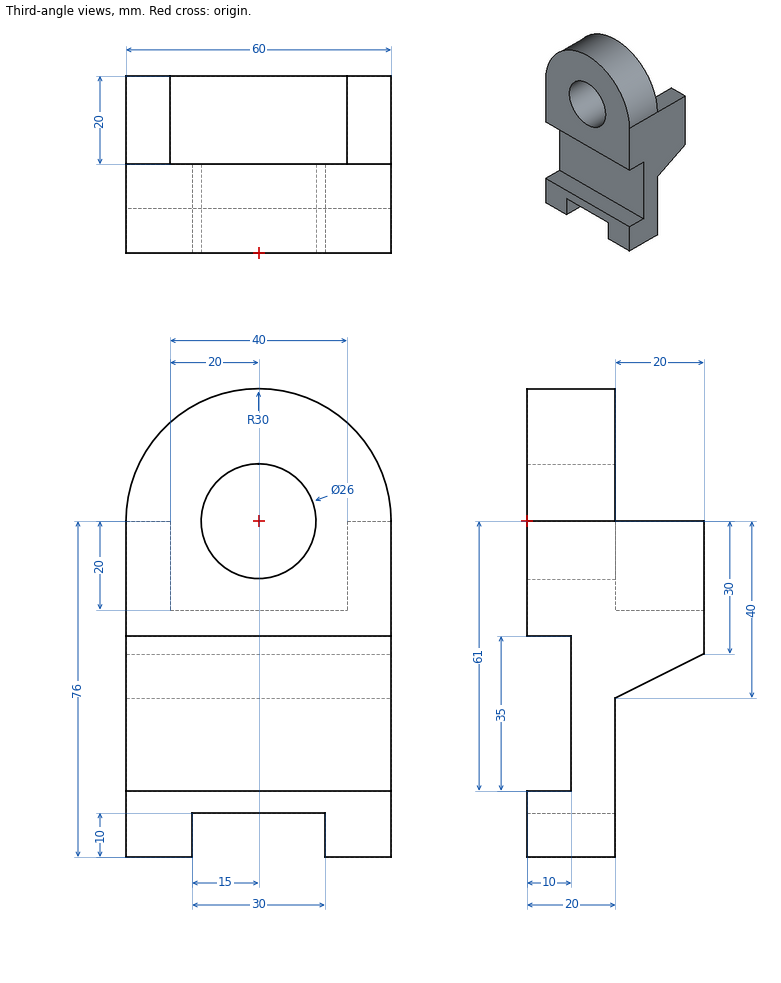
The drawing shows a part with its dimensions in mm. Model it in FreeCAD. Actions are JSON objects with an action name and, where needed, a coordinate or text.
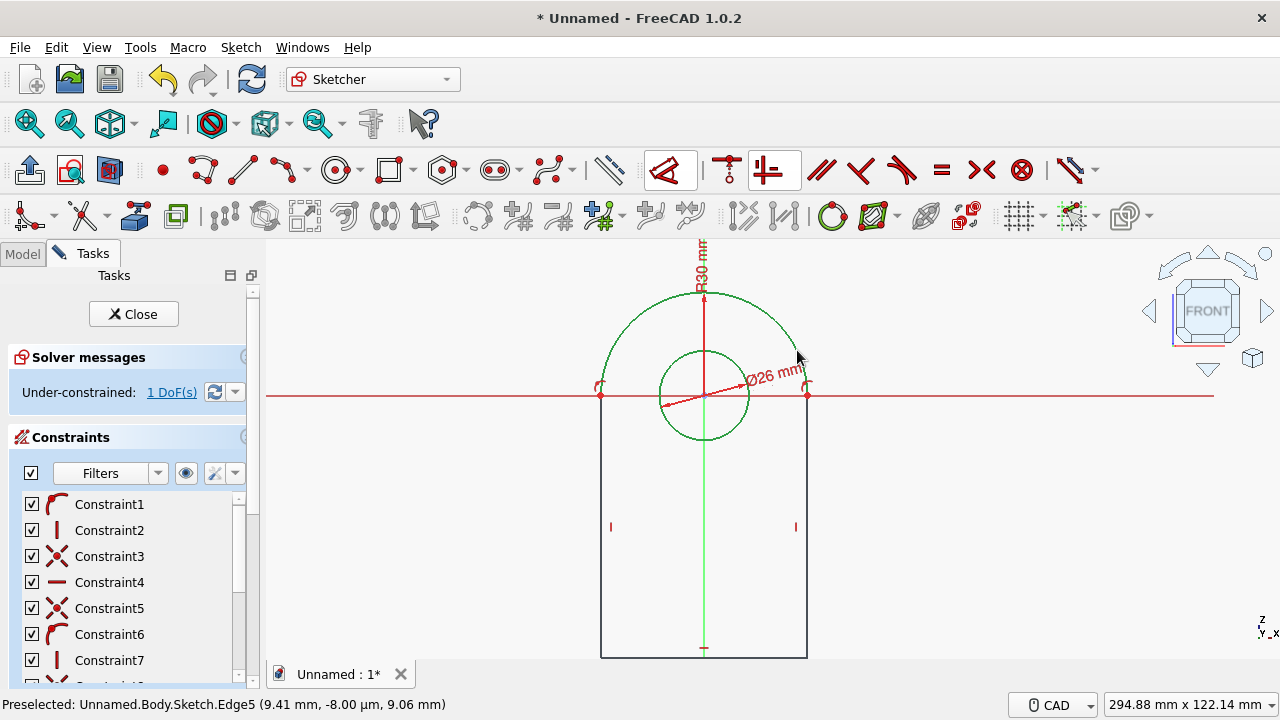
{"action": "left_click", "coordinate": [601, 474]}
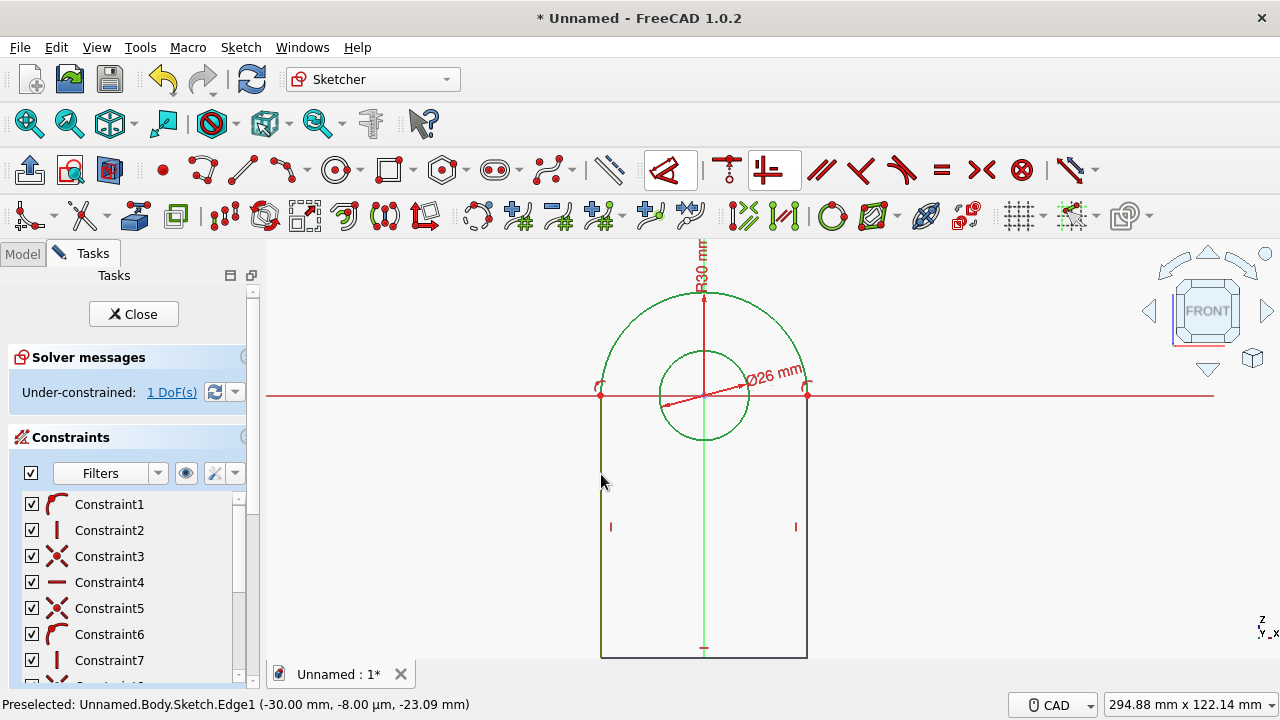
{"action": "key", "text": "i"}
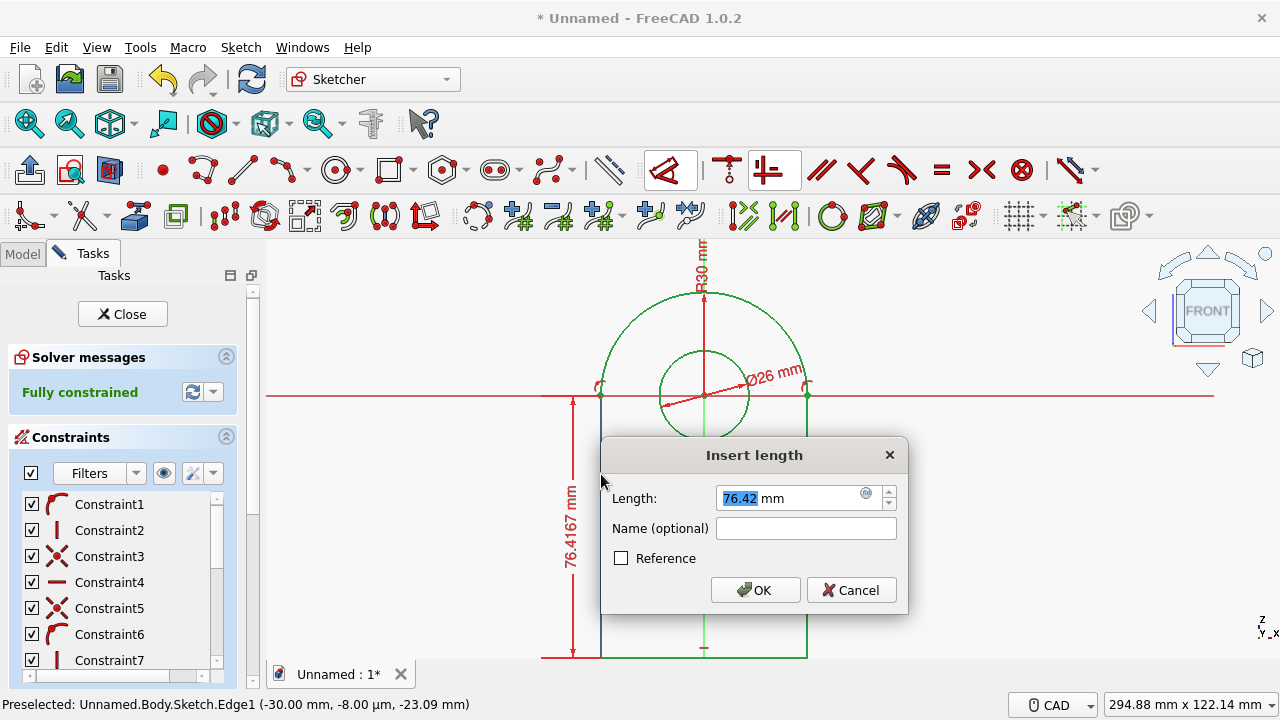
{"action": "type", "text": "76"}
{"action": "key", "text": "Return"}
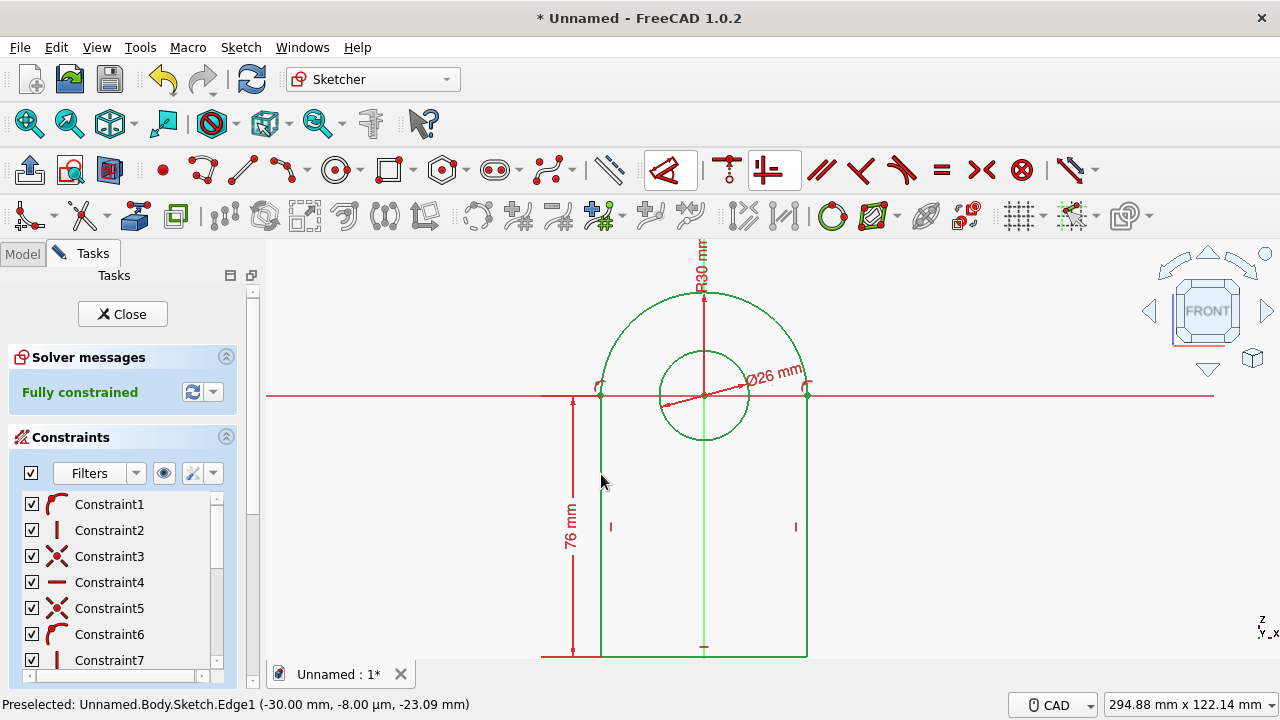
{"action": "left_click", "coordinate": [123, 314]}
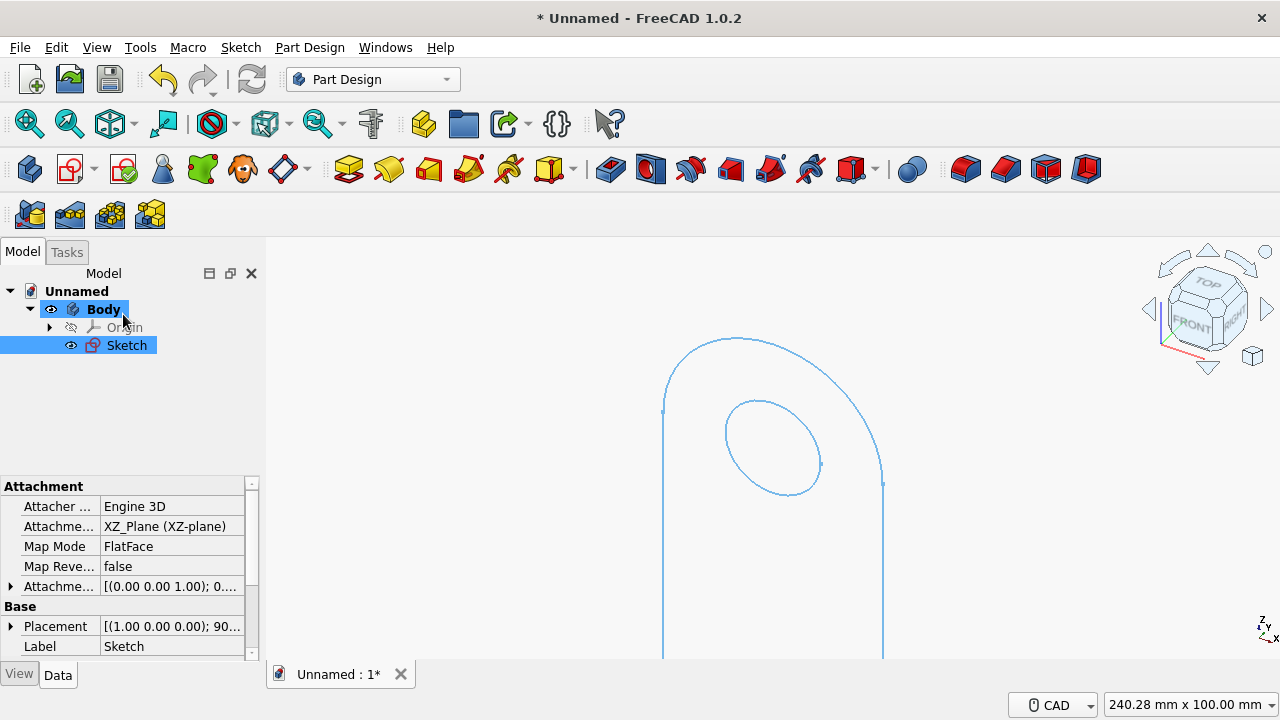
{"action": "left_click", "coordinate": [350, 170]}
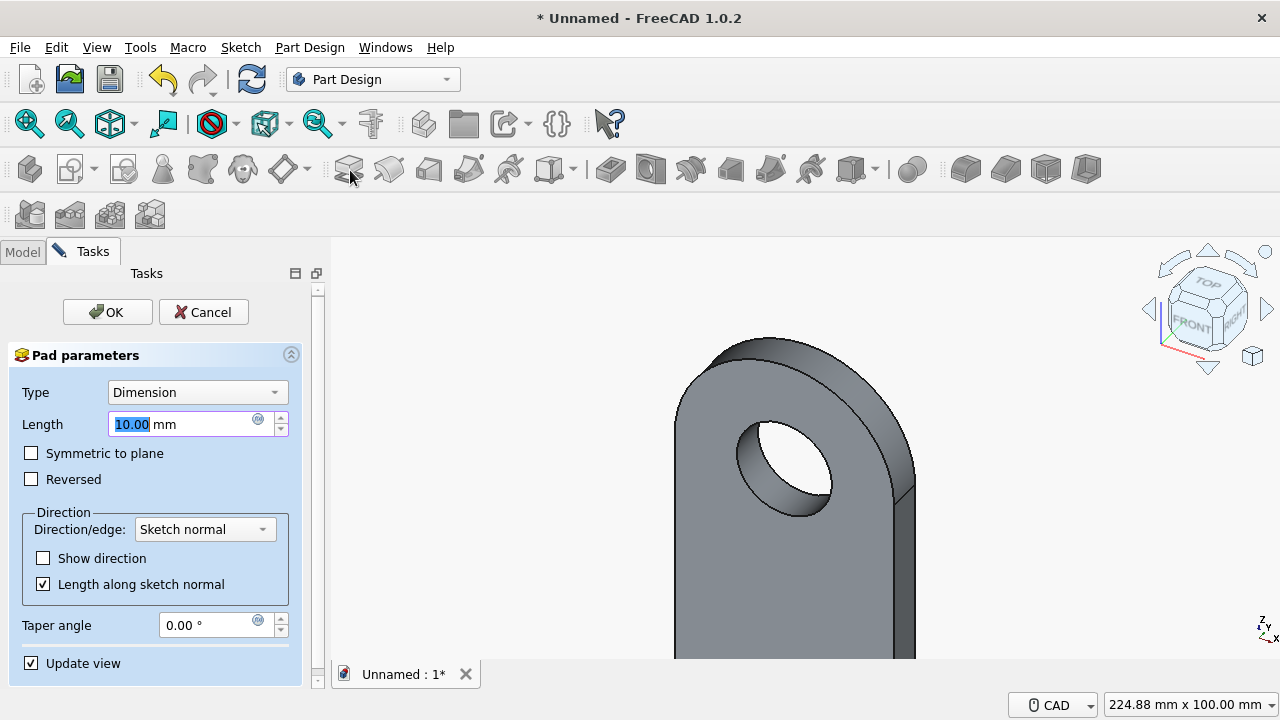
{"action": "type", "text": "20"}
{"action": "key", "text": "Tab"}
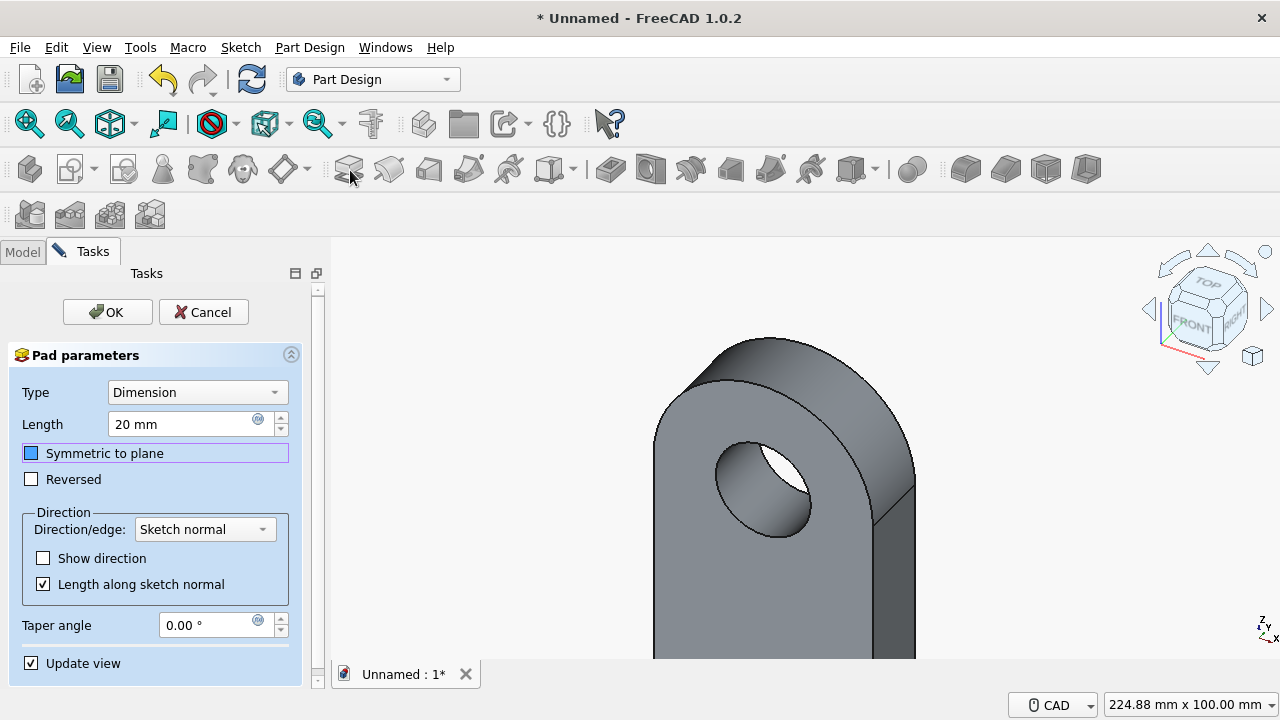
{"action": "left_click", "coordinate": [30, 479]}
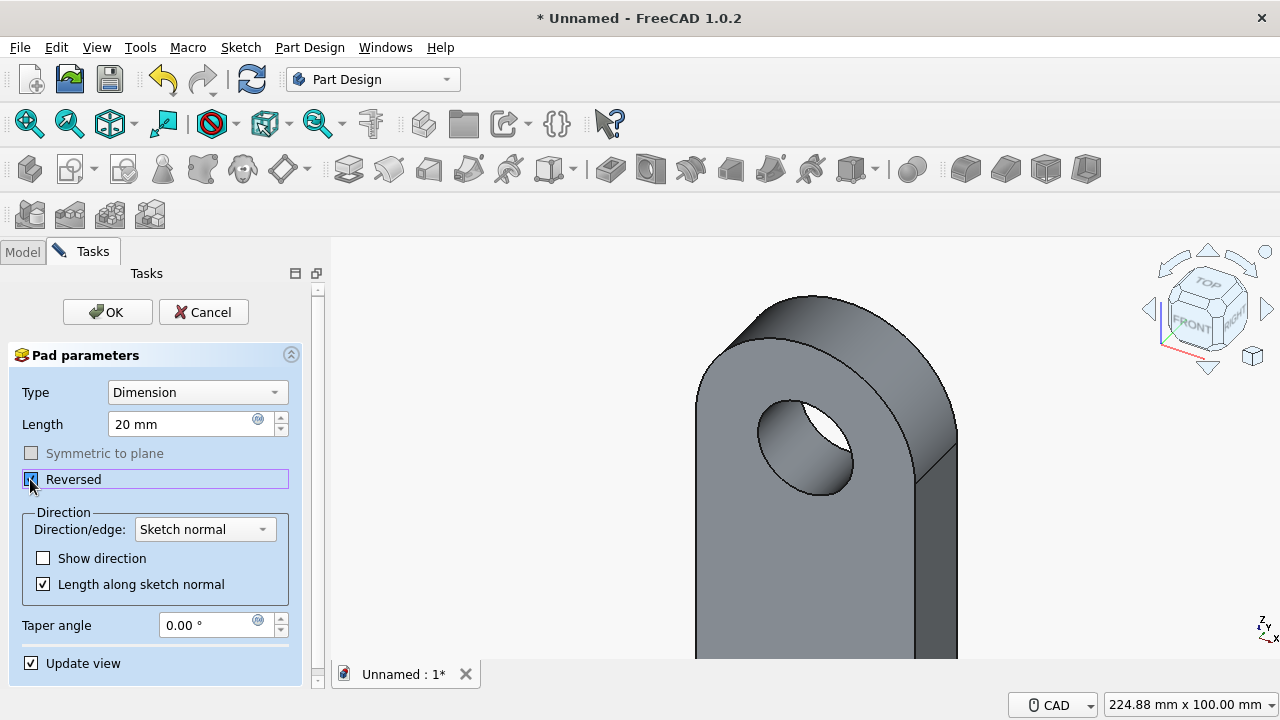
{"action": "left_click", "coordinate": [108, 312]}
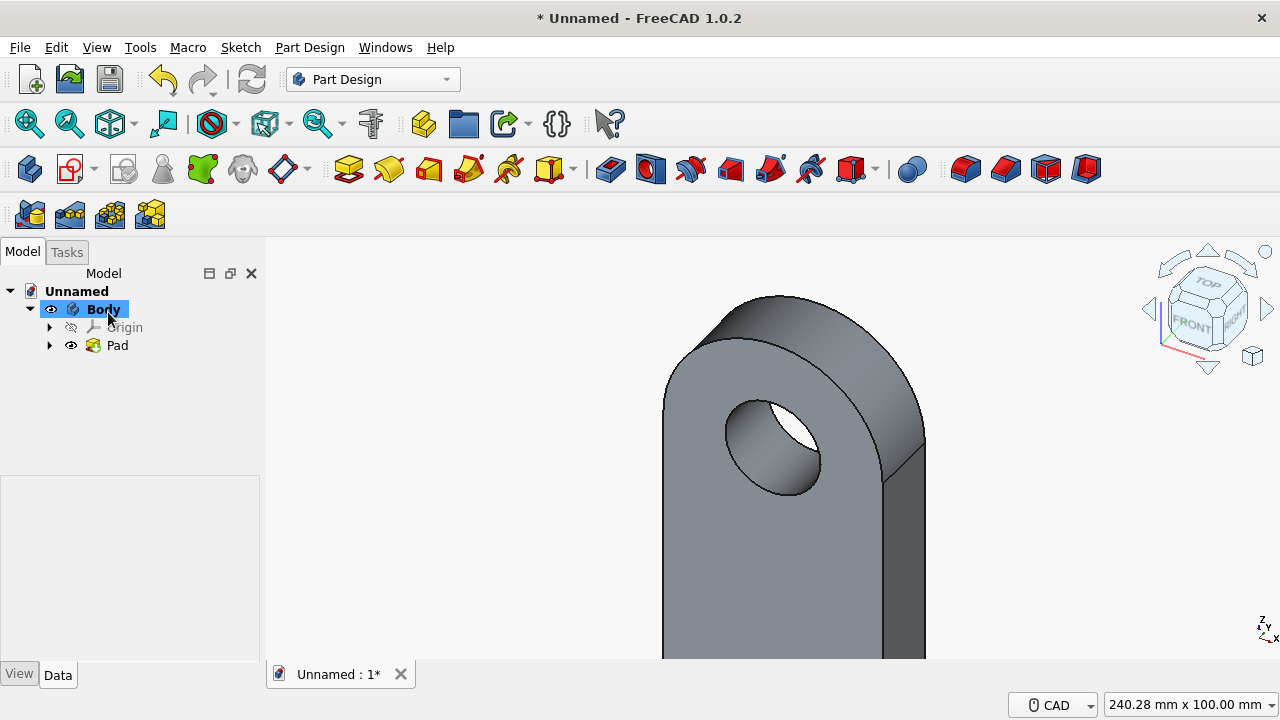
{"action": "key", "text": "v f"}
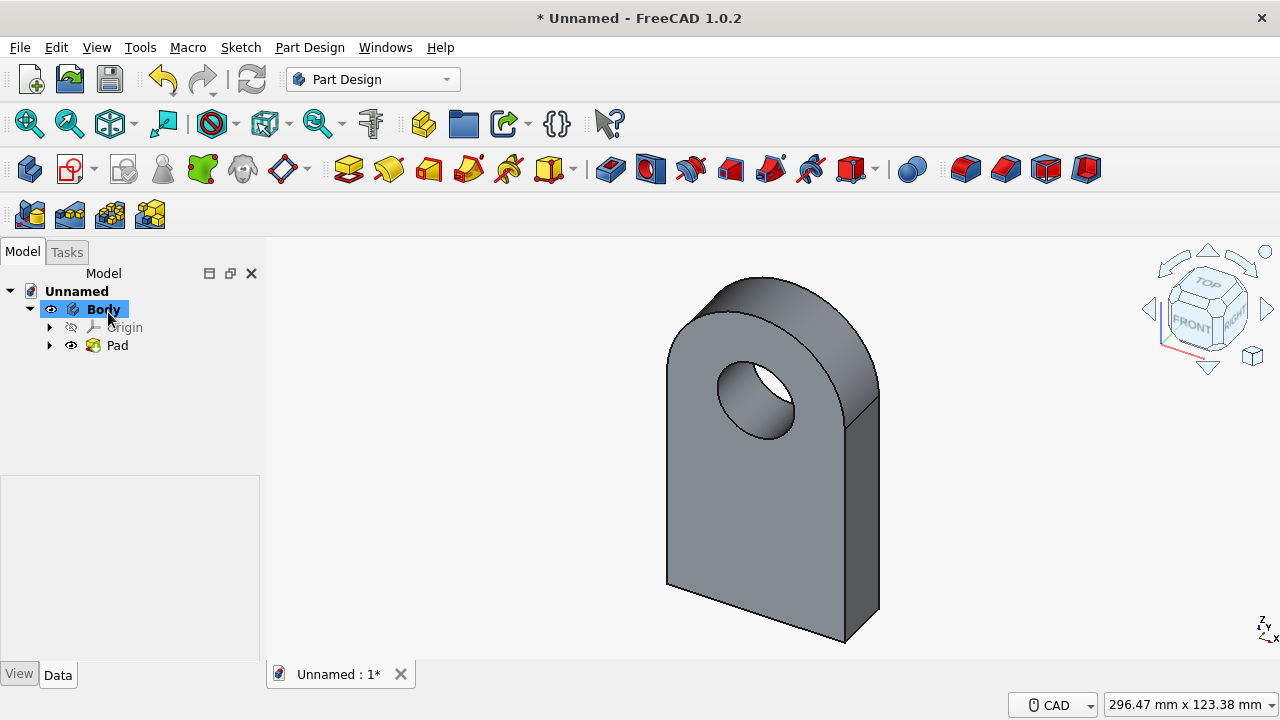
{"action": "left_click", "coordinate": [862, 458]}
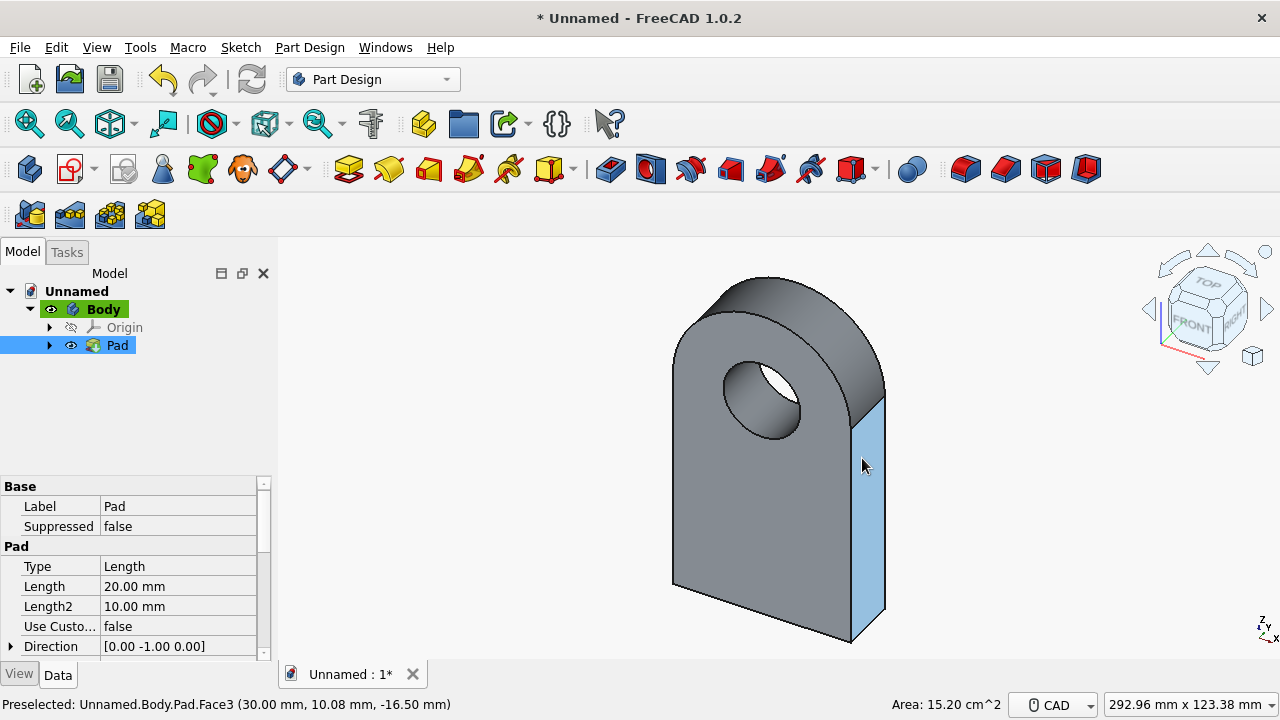
{"action": "left_click", "coordinate": [70, 170]}